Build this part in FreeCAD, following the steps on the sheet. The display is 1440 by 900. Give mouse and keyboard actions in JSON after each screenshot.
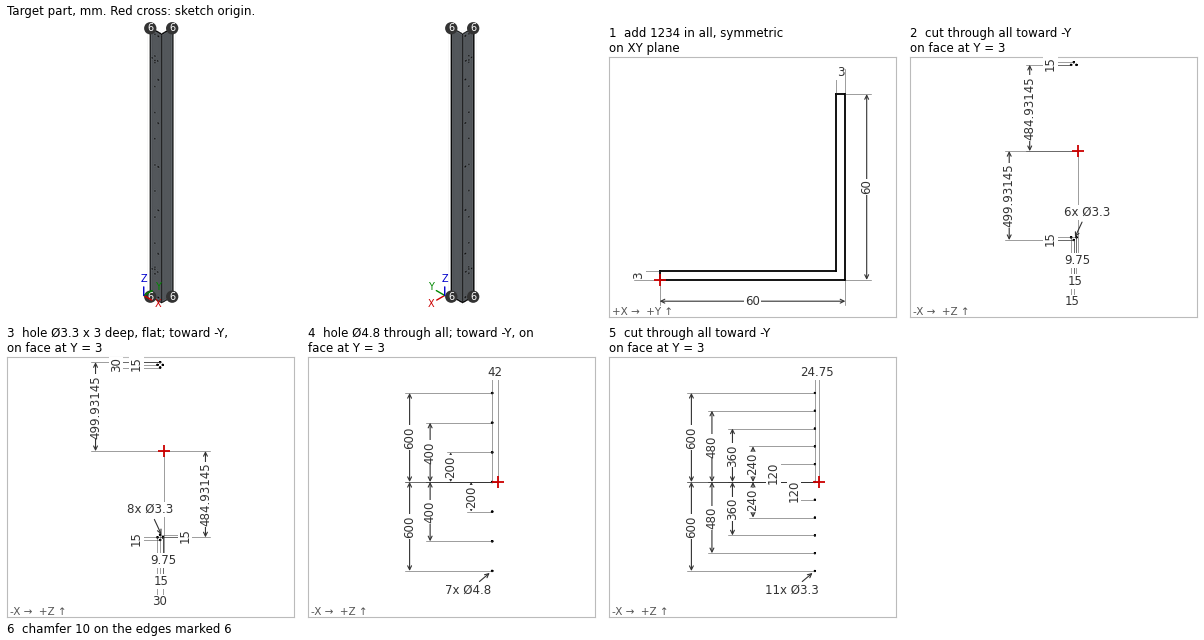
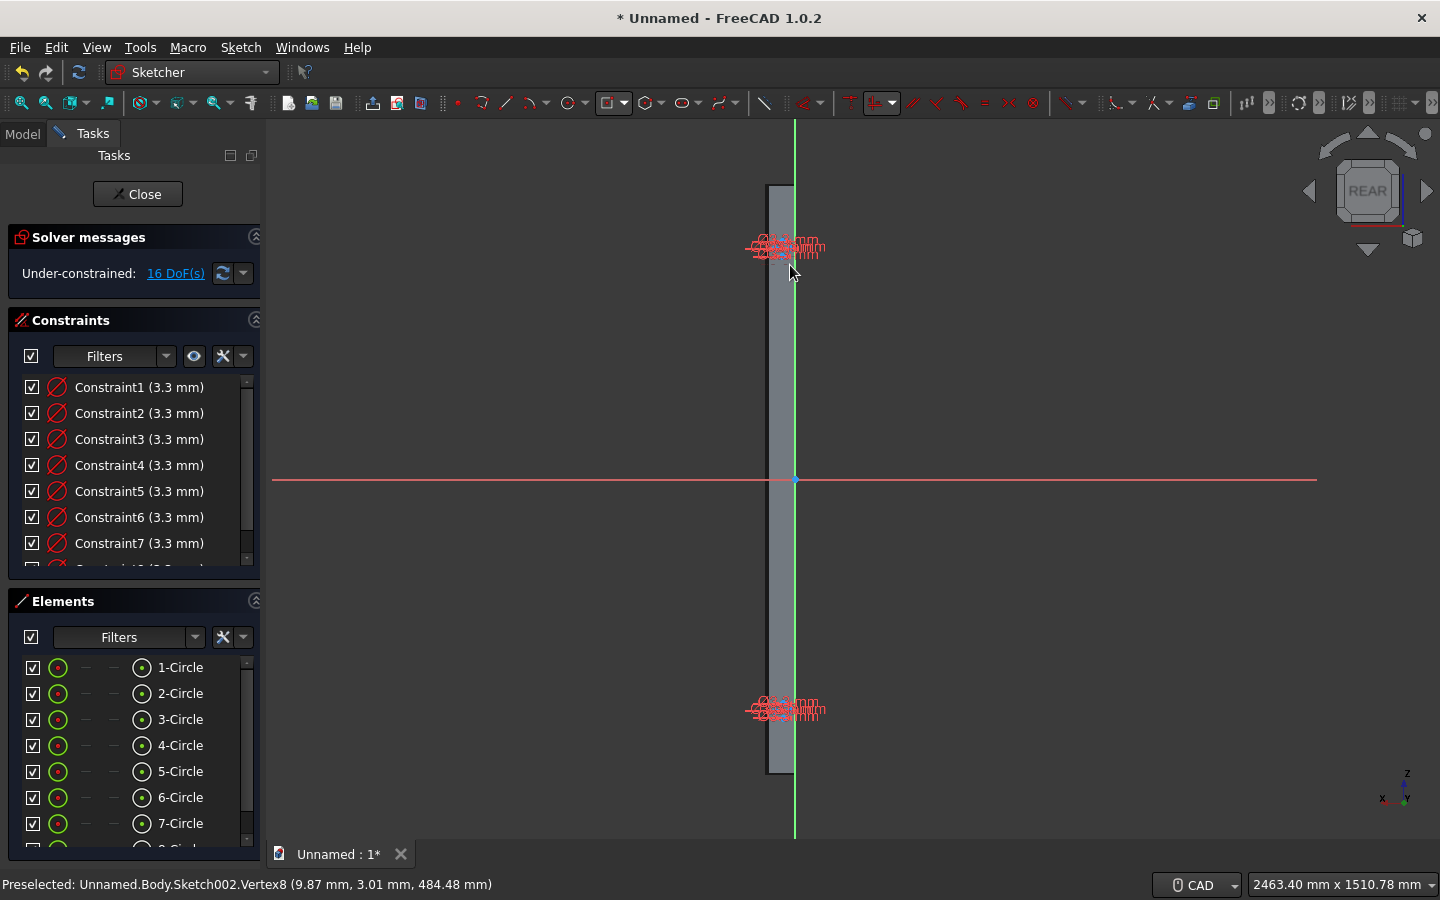
{"action": "left_click", "coordinate": [791, 711]}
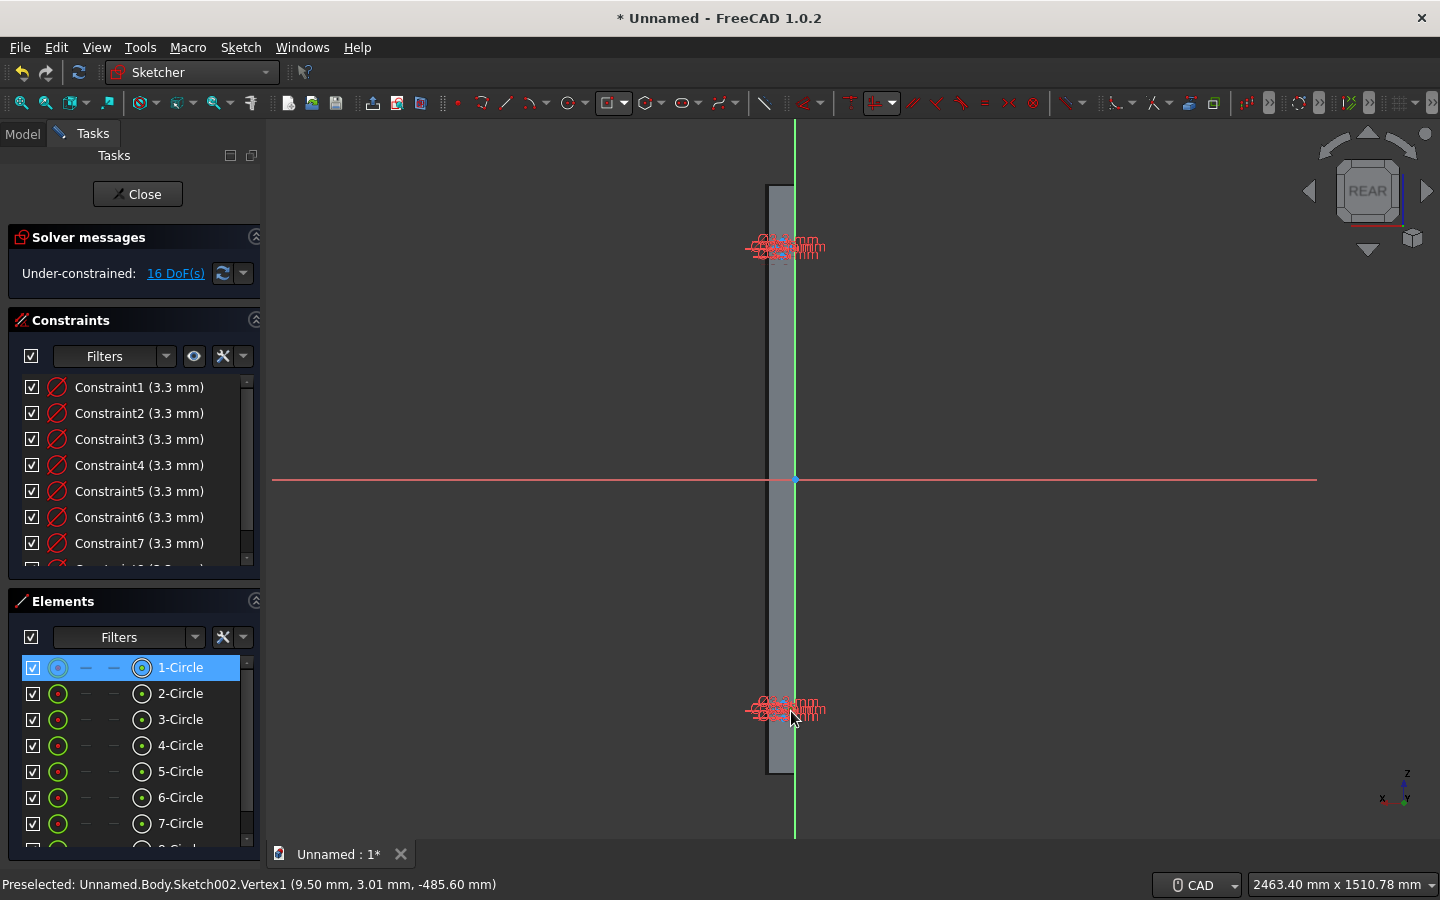
{"action": "left_click", "coordinate": [776, 711]}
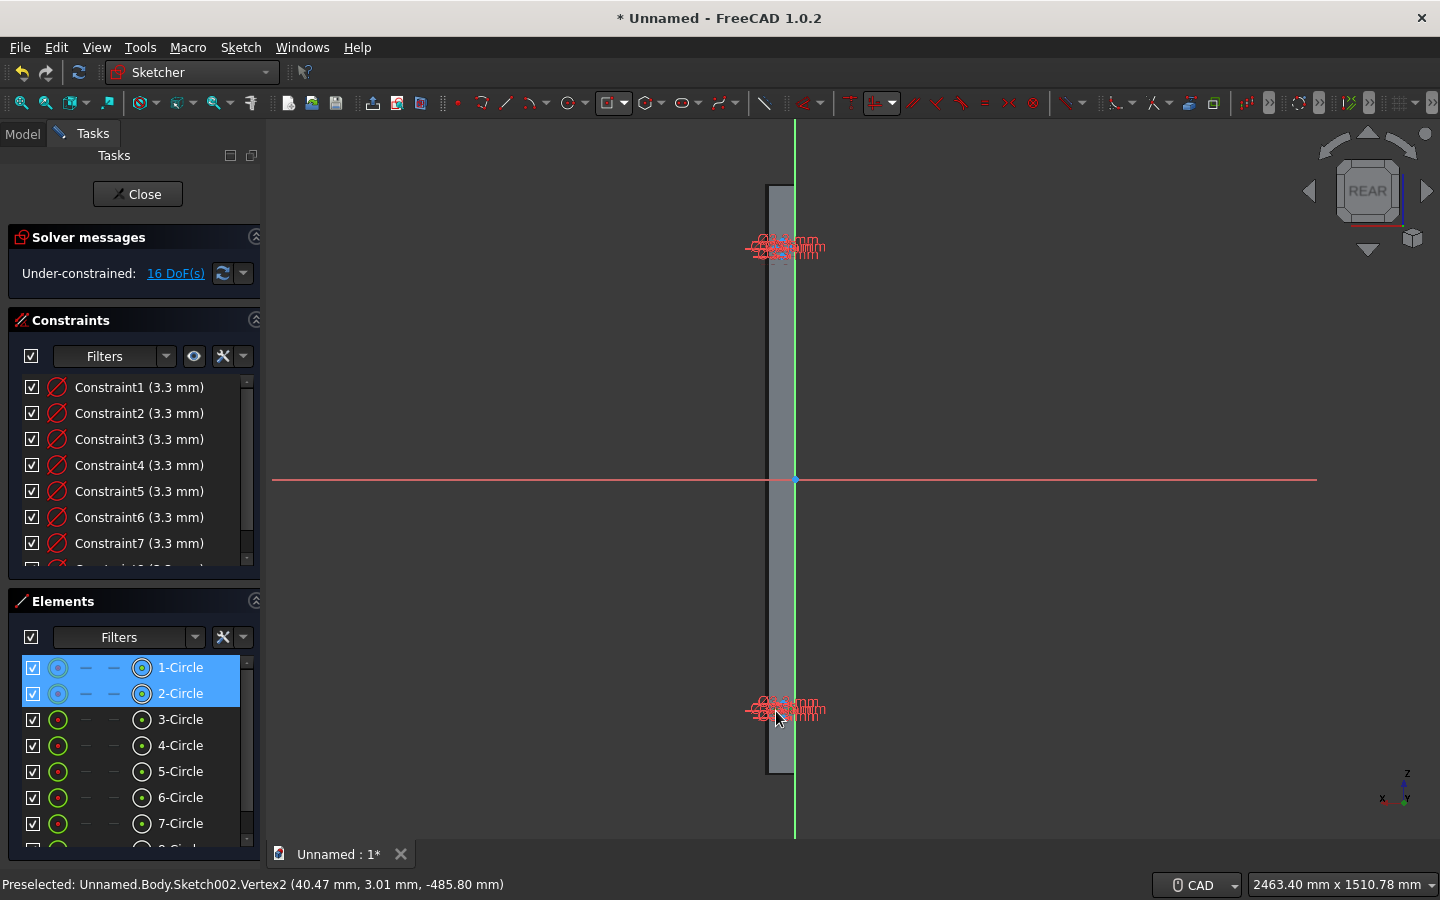
{"action": "left_click", "coordinate": [894, 104]}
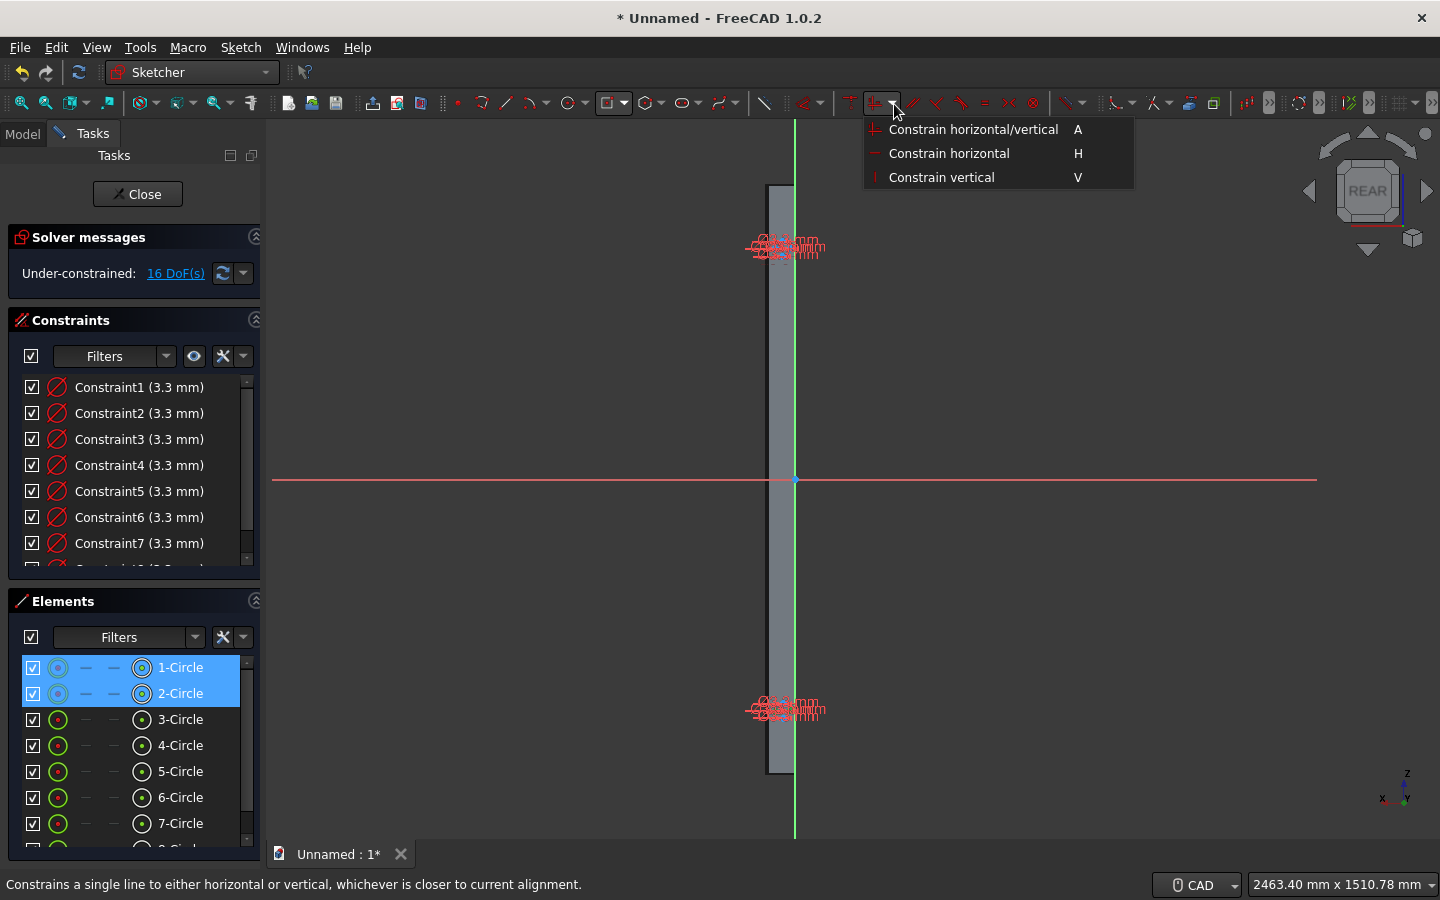
{"action": "left_click", "coordinate": [999, 153]}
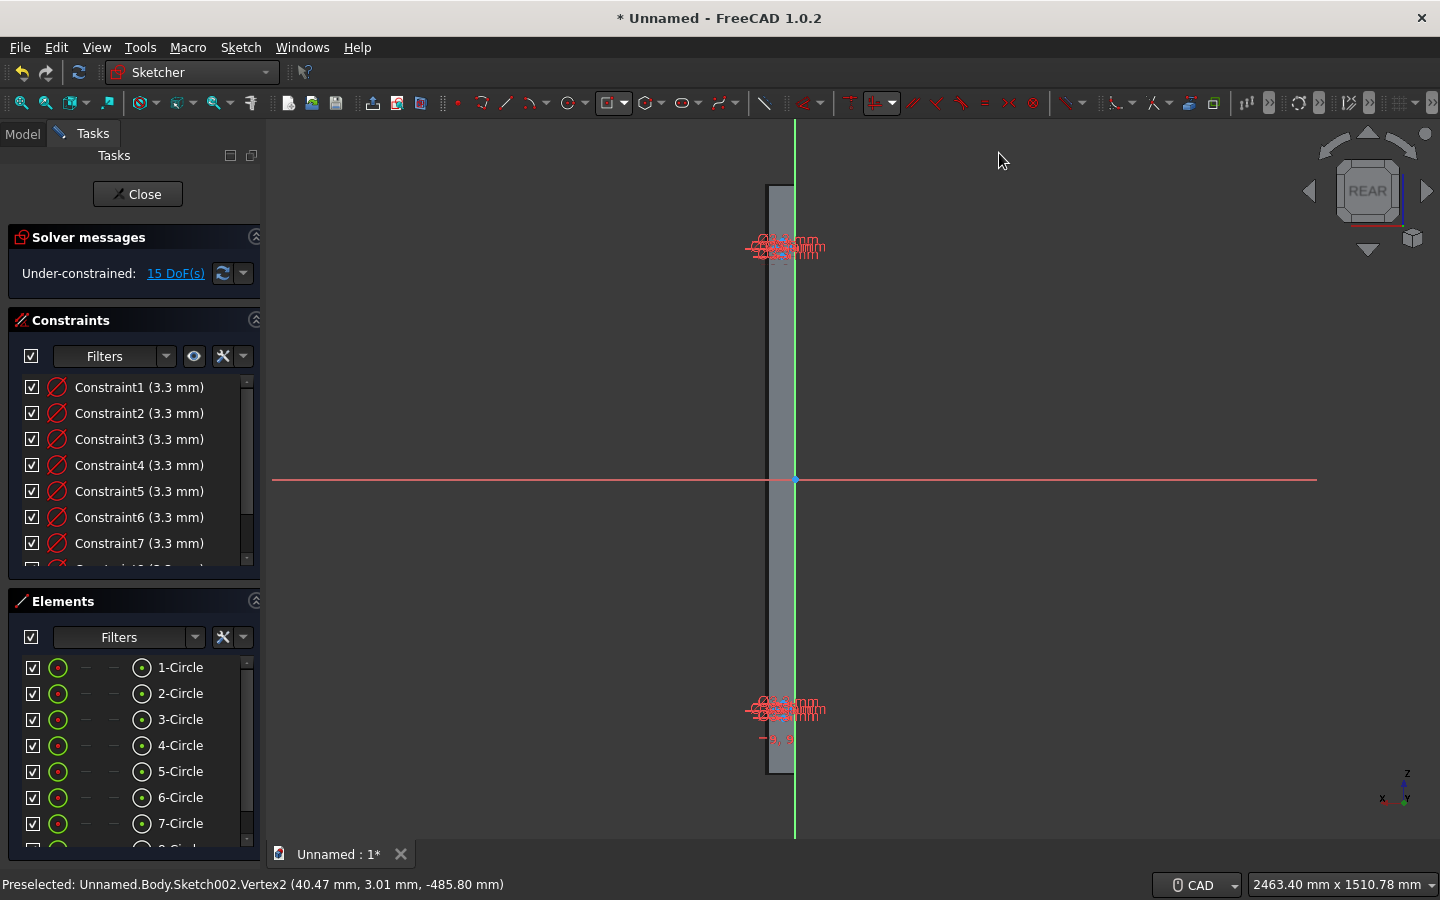
{"action": "left_click", "coordinate": [783, 704]}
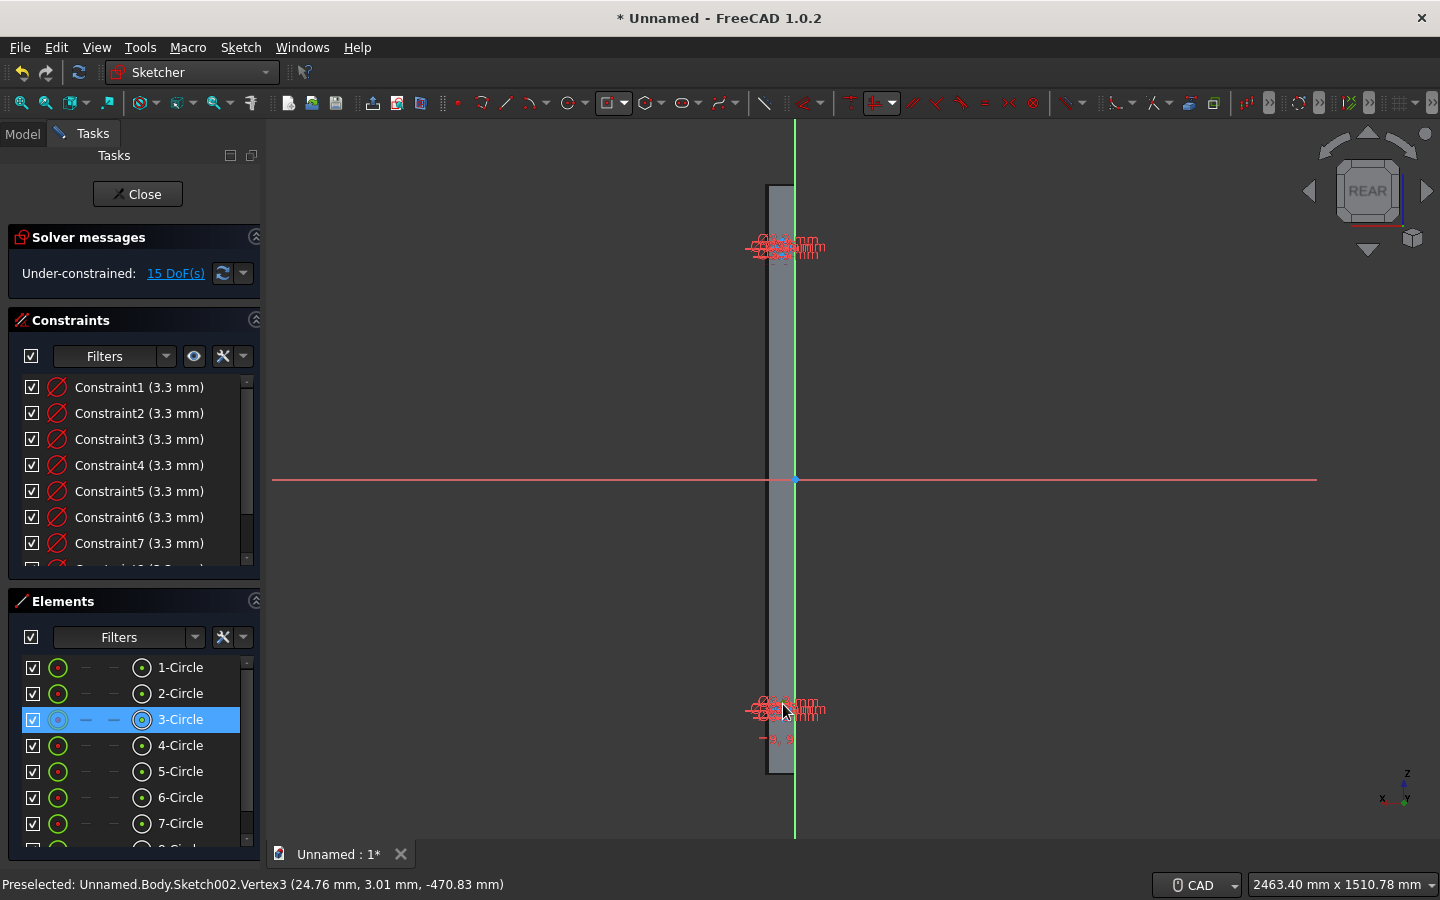
{"action": "left_click", "coordinate": [783, 718]}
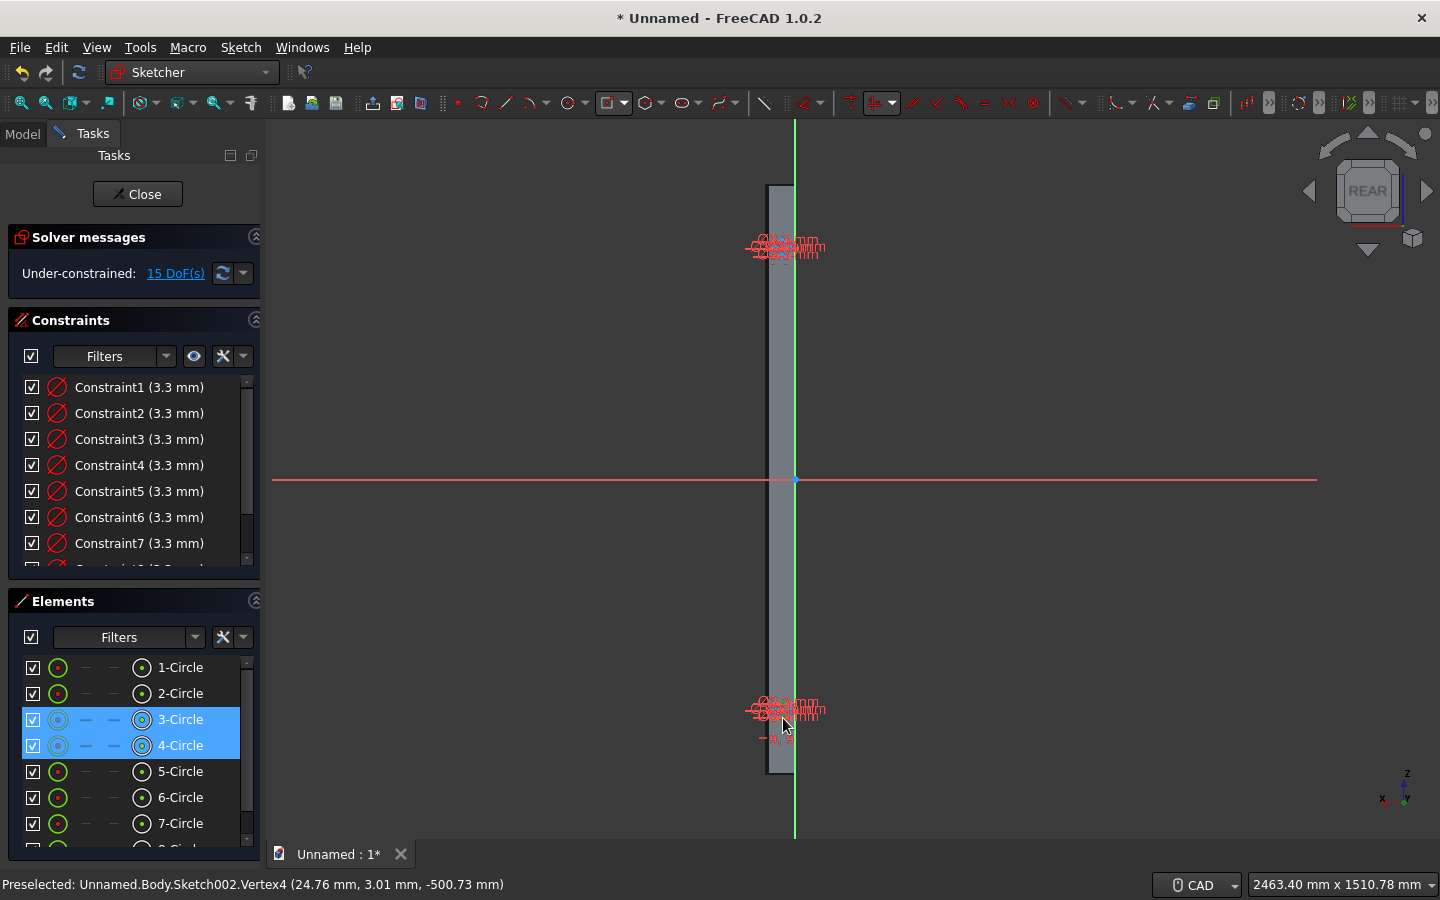
{"action": "key", "text": "v"}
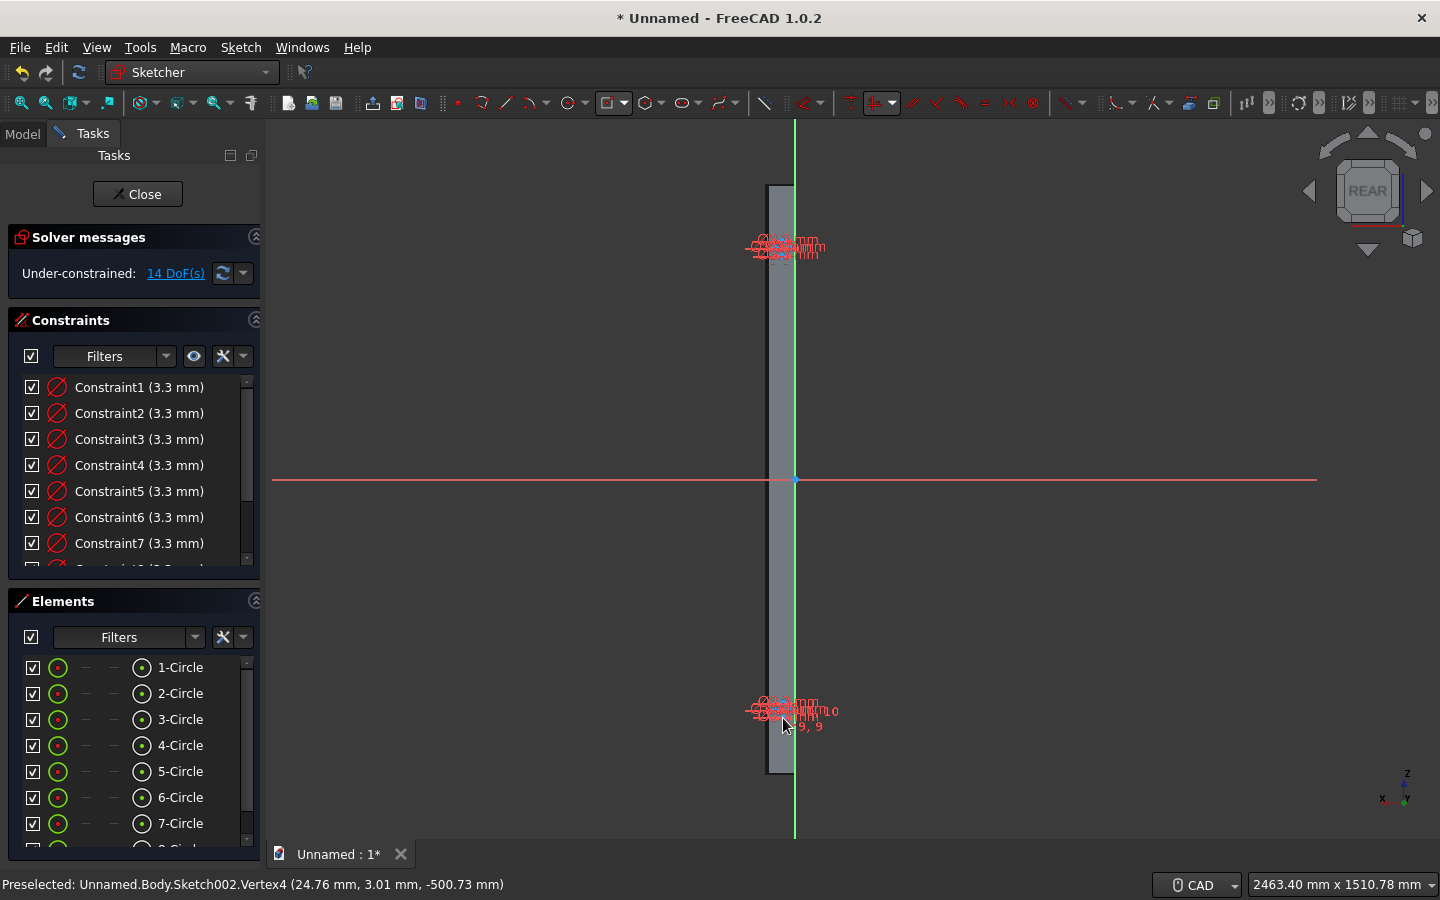
{"action": "left_click", "coordinate": [783, 704]}